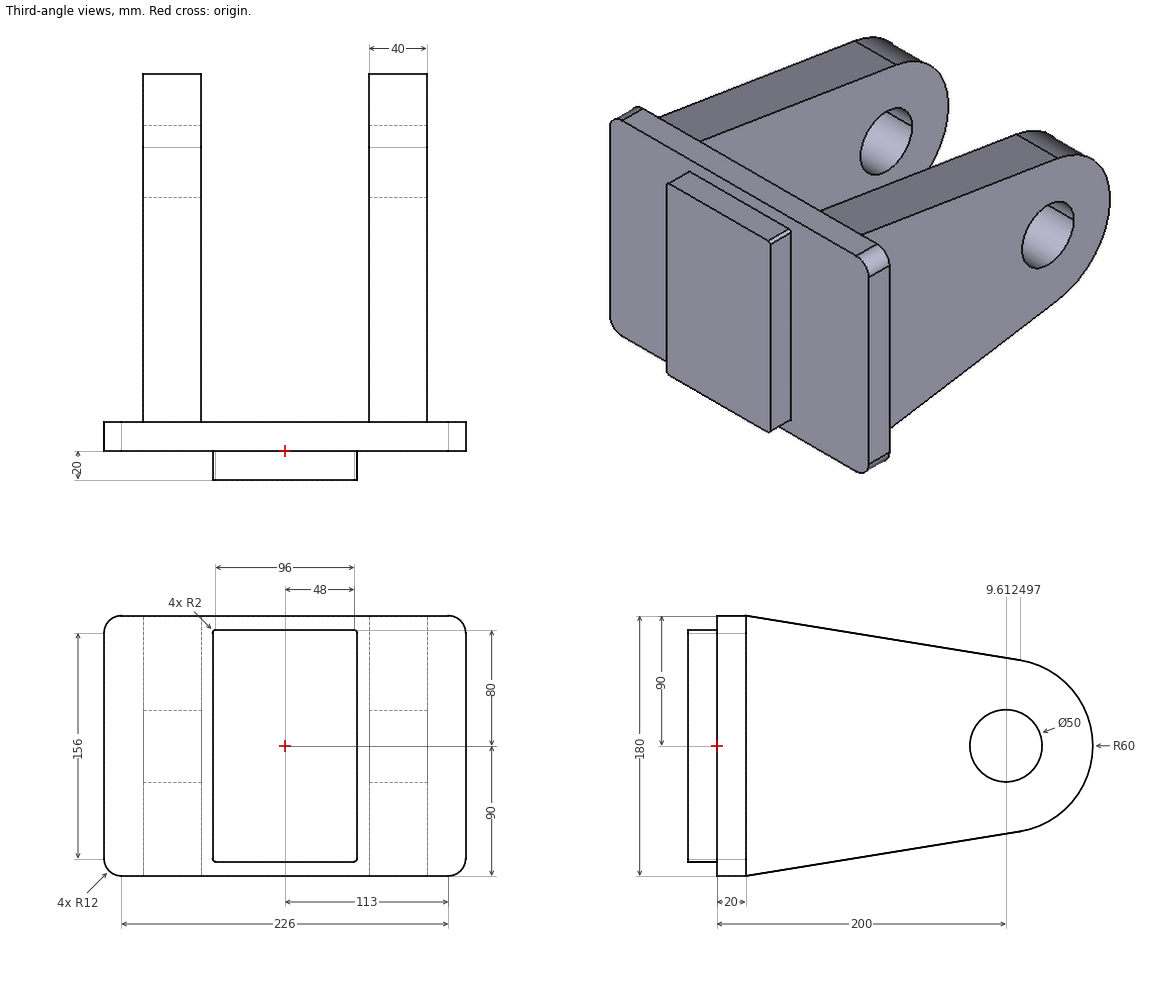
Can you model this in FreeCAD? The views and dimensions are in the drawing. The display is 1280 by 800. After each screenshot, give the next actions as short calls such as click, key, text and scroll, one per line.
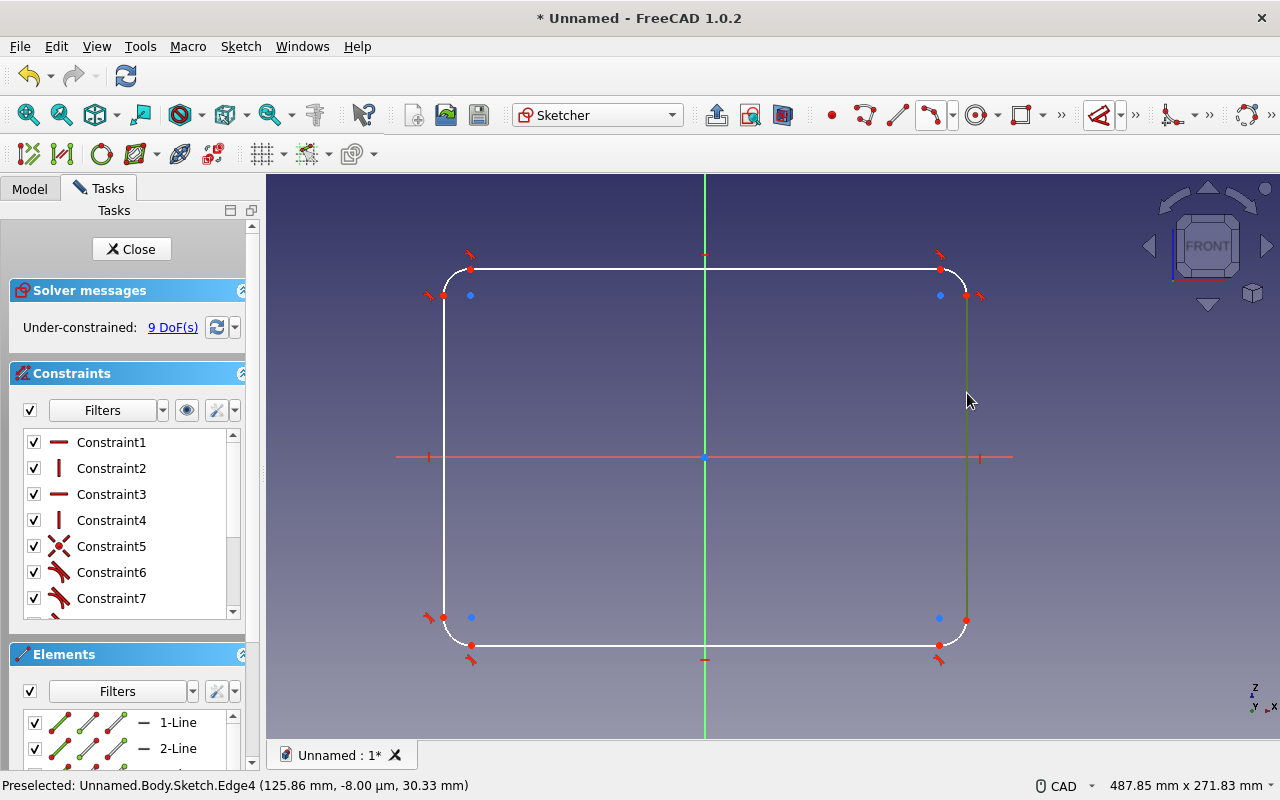
click(951, 643)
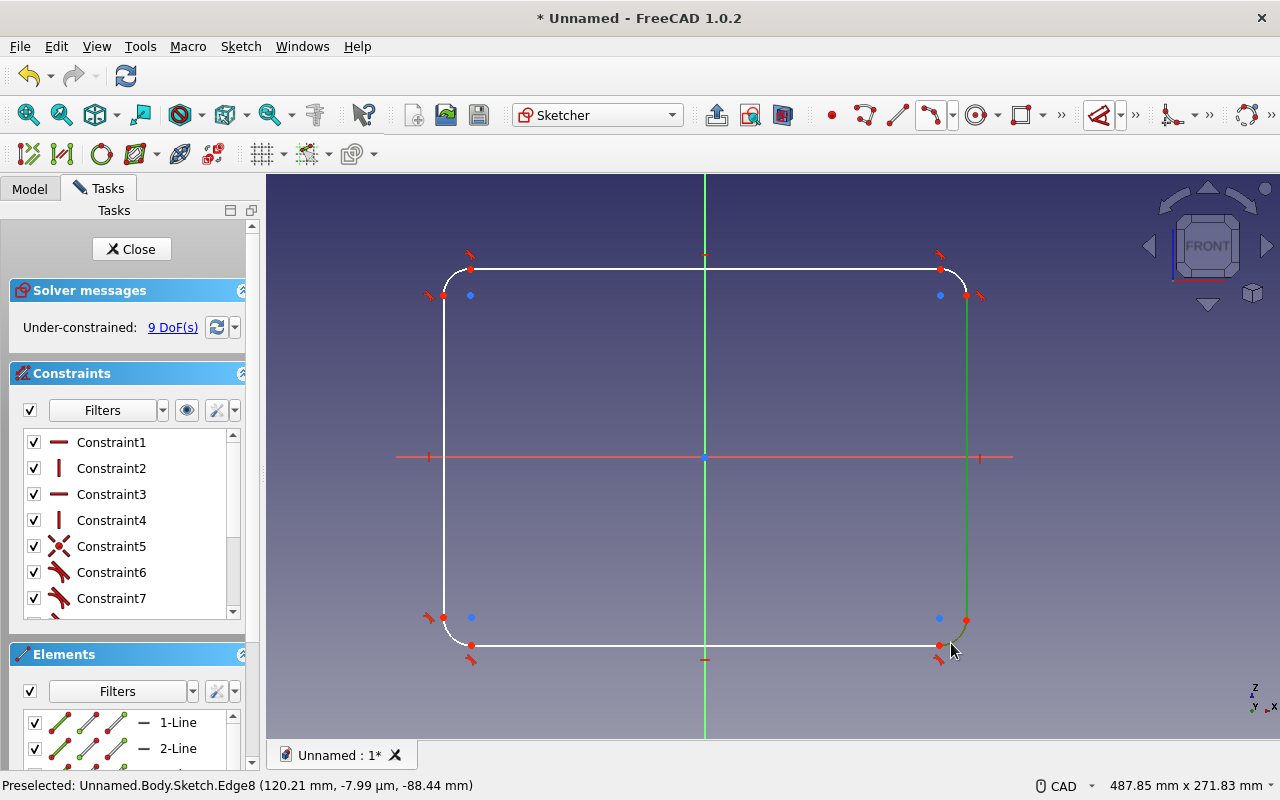
key(t)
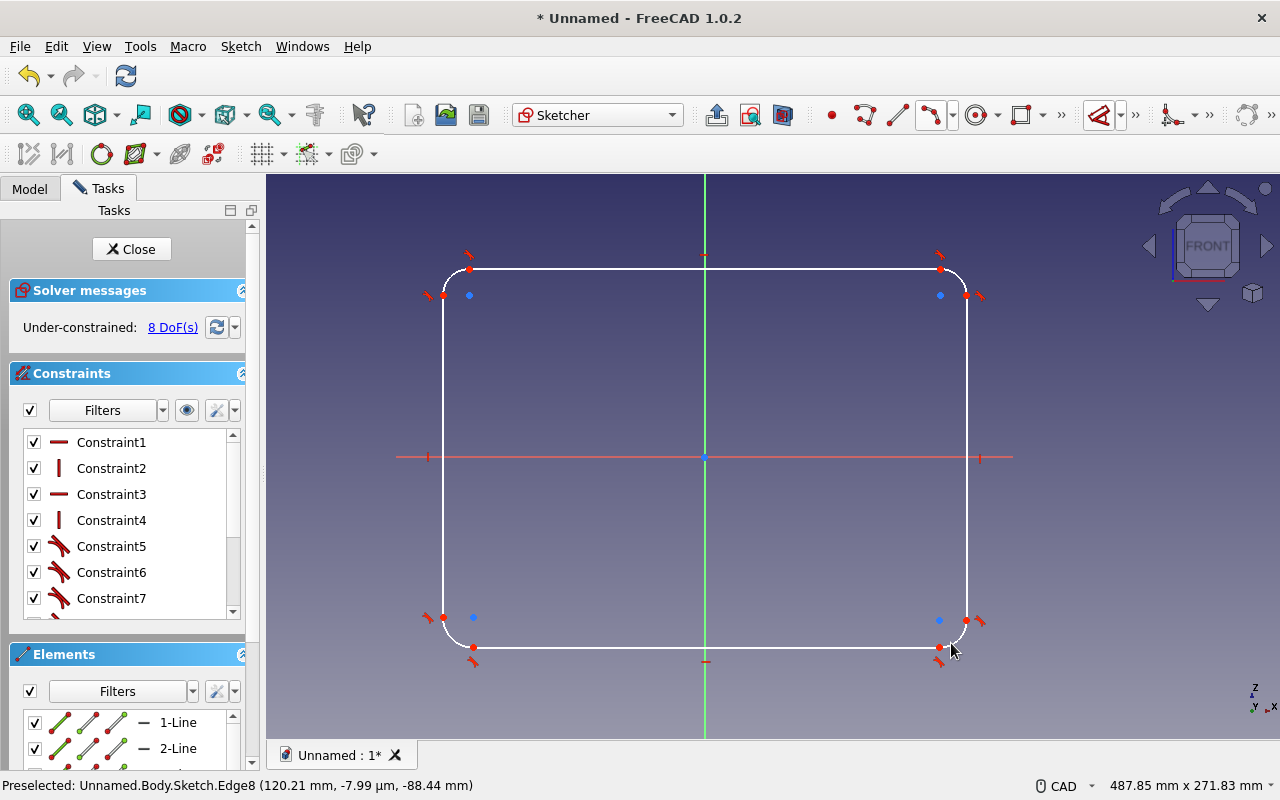
click(446, 631)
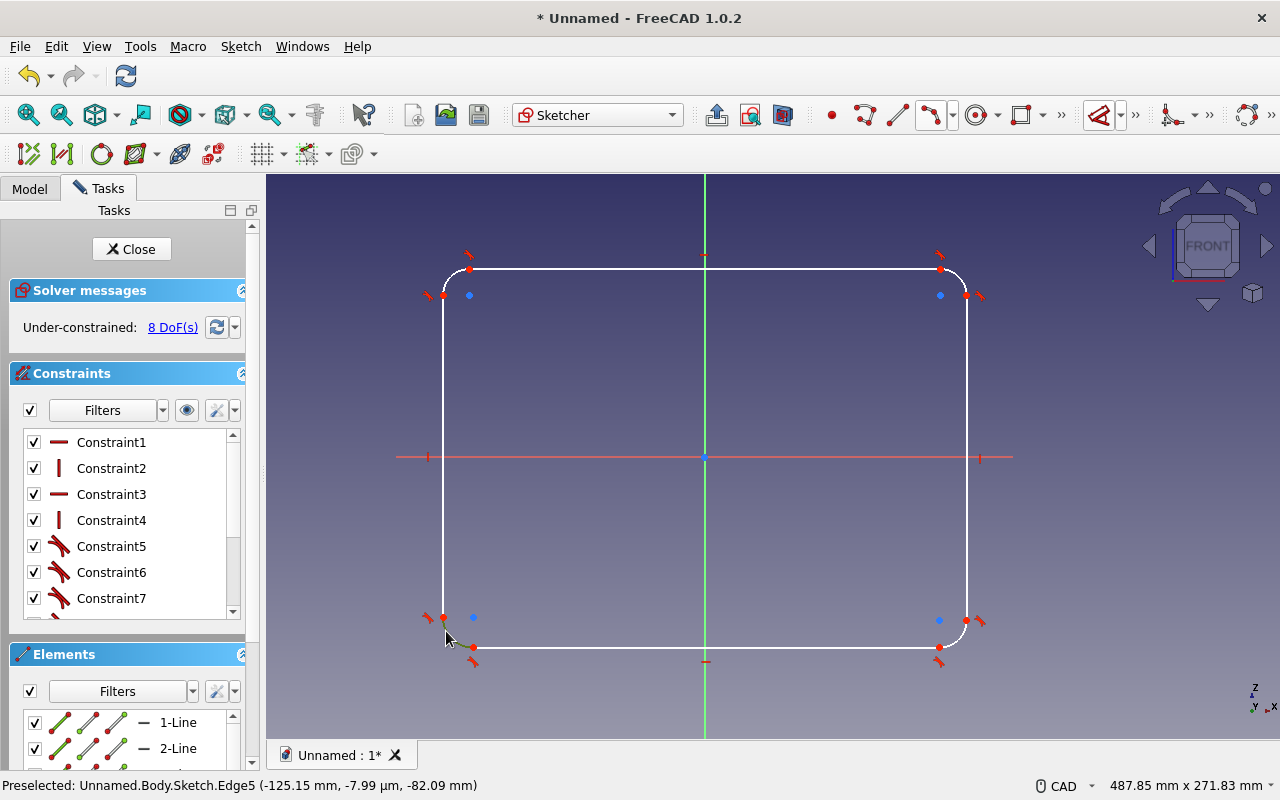
click(457, 272)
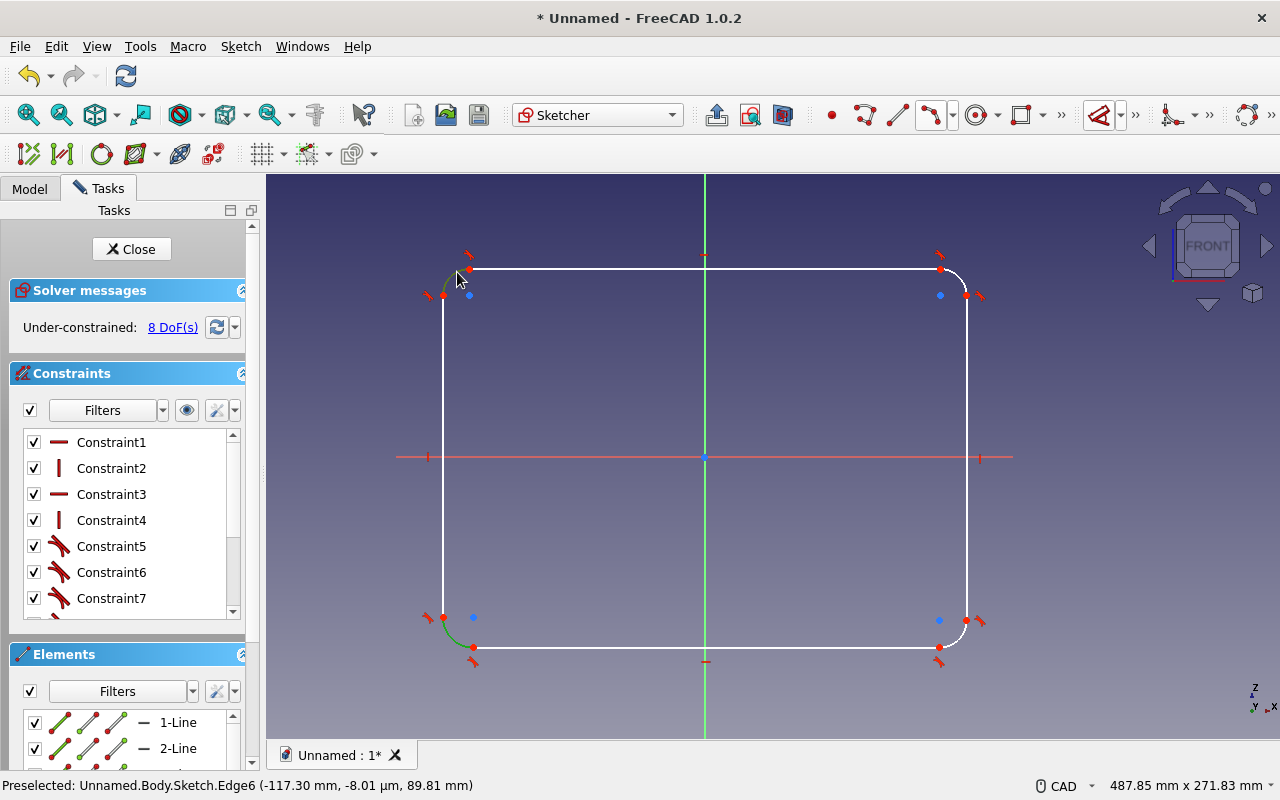
click(964, 284)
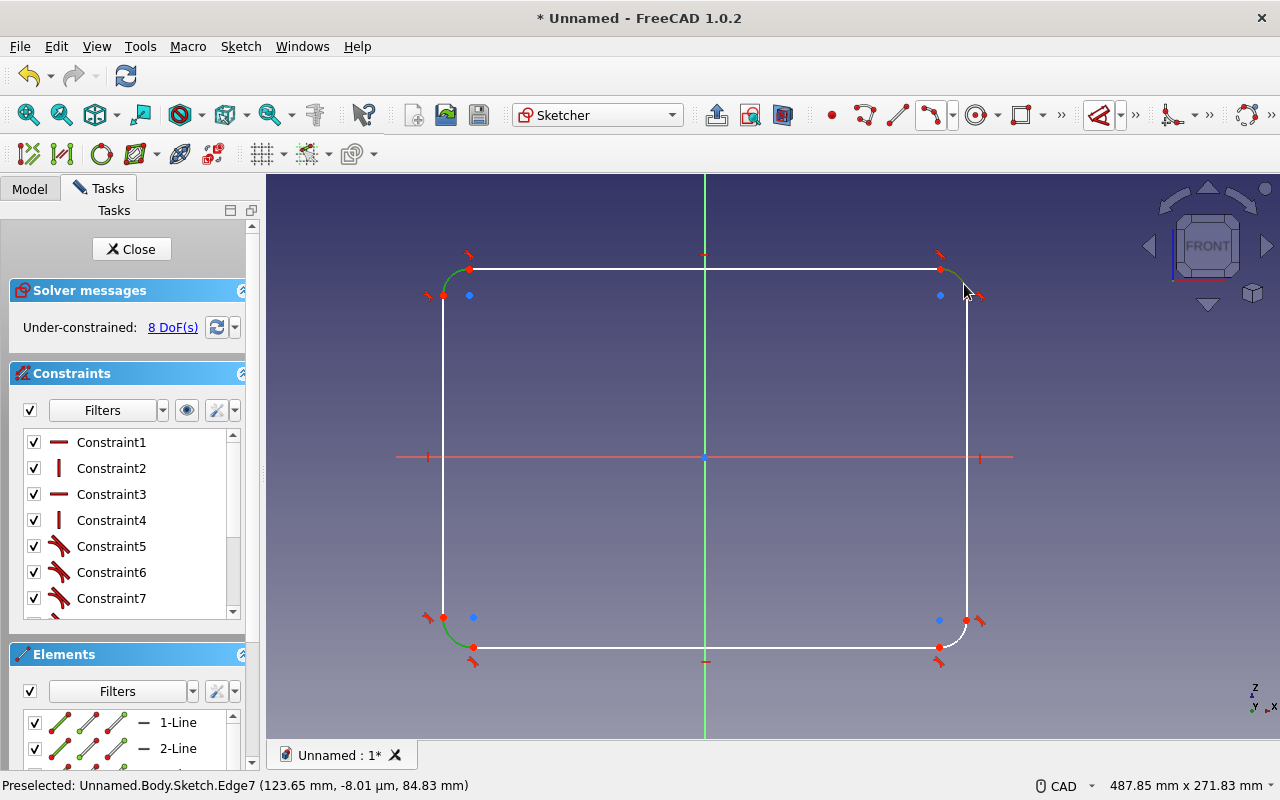
click(952, 645)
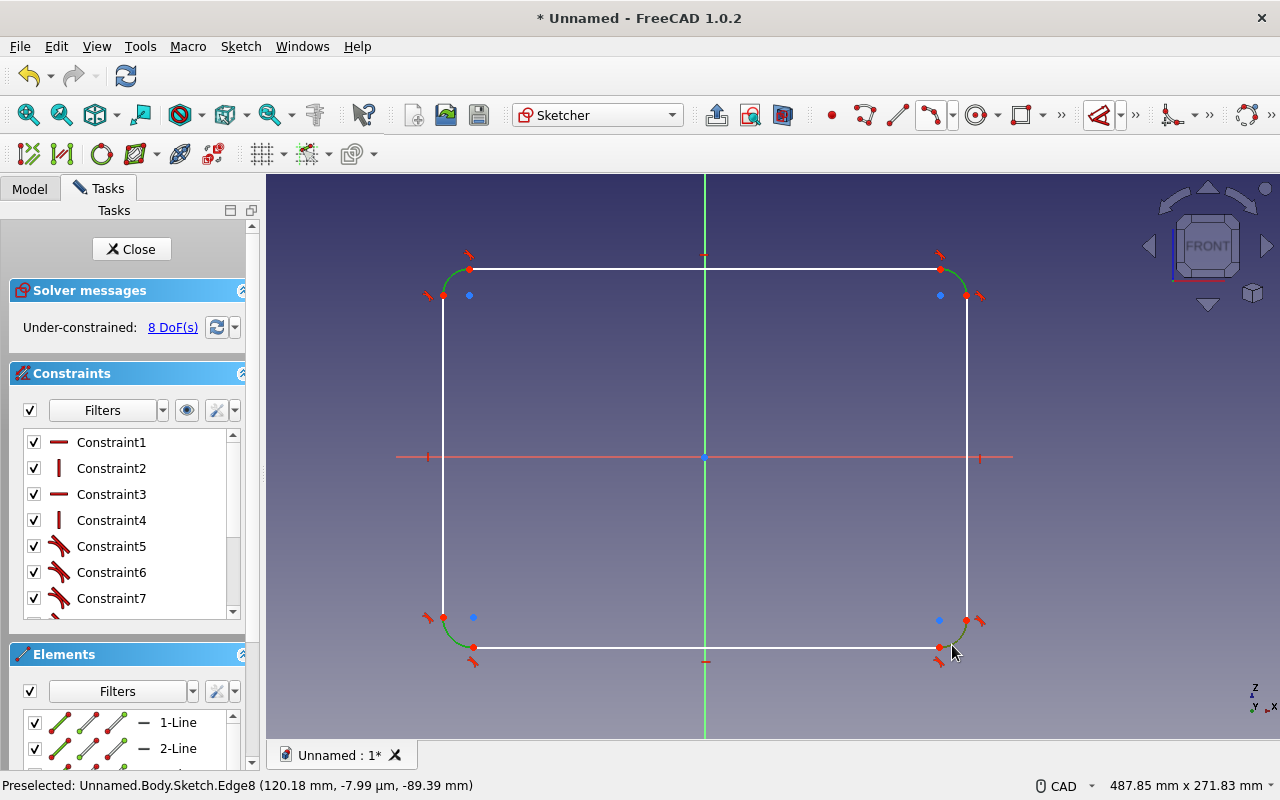
key(e)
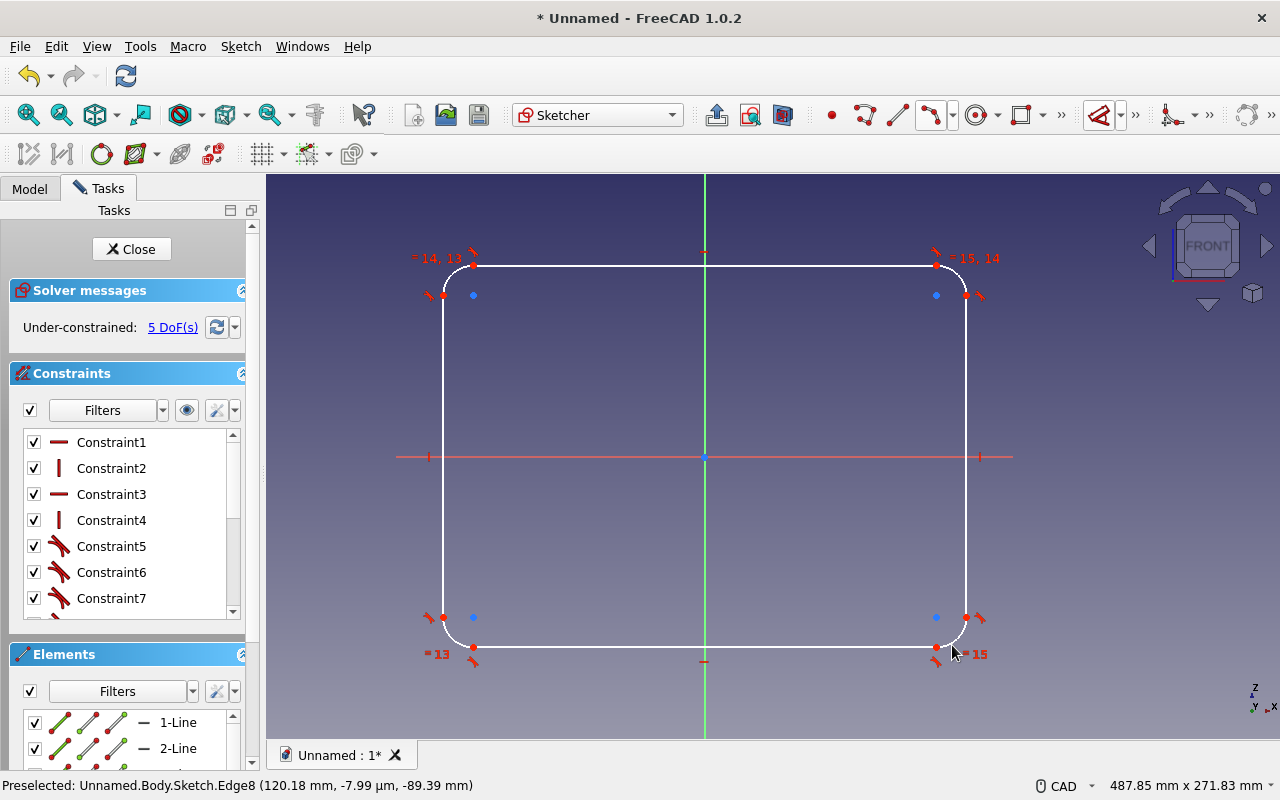
click(1098, 116)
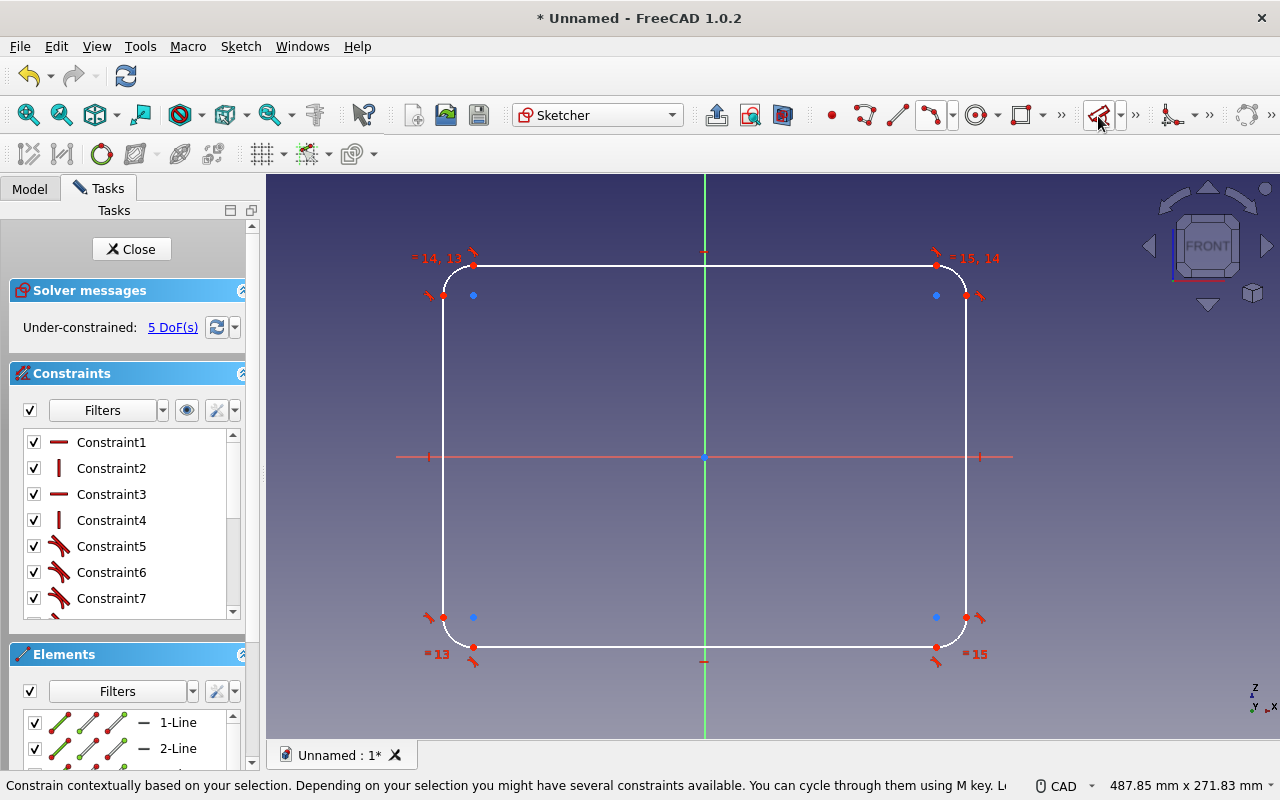
scroll(446, 631, up, 3)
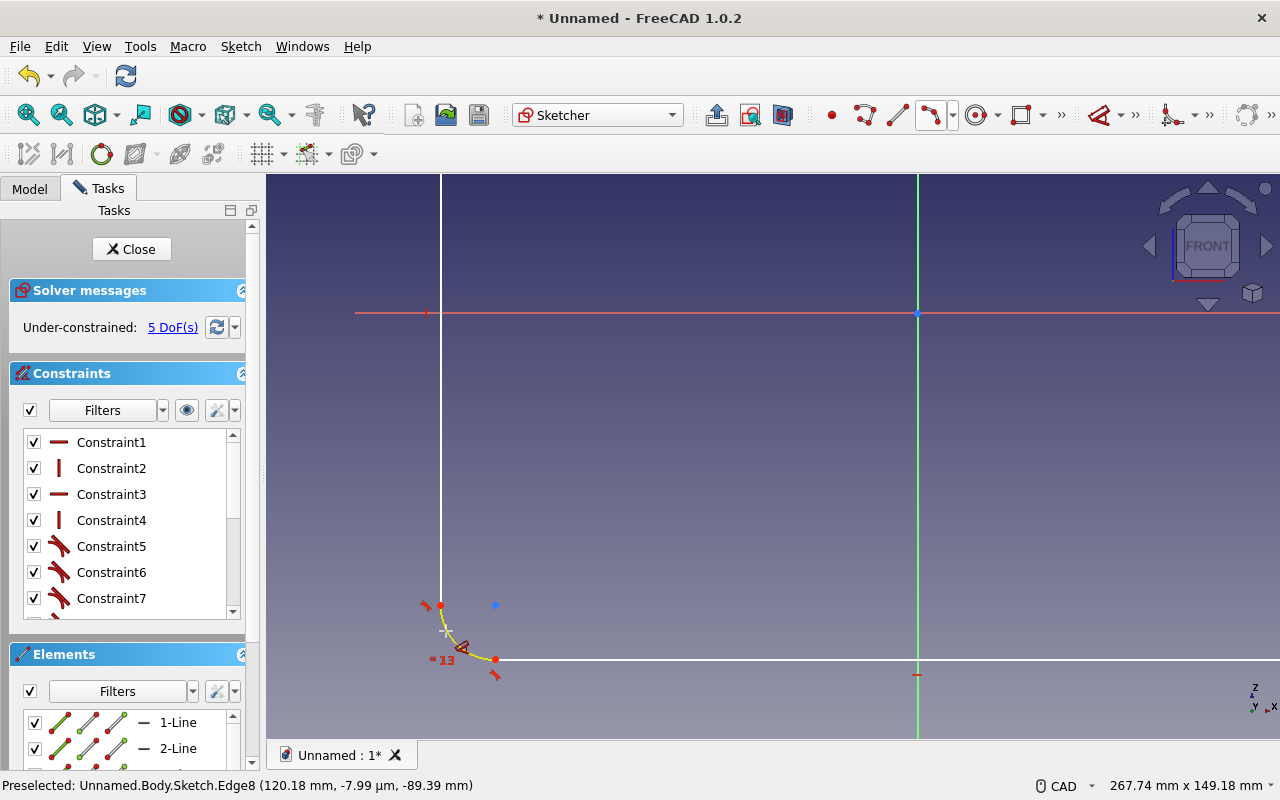
click(447, 630)
click(418, 644)